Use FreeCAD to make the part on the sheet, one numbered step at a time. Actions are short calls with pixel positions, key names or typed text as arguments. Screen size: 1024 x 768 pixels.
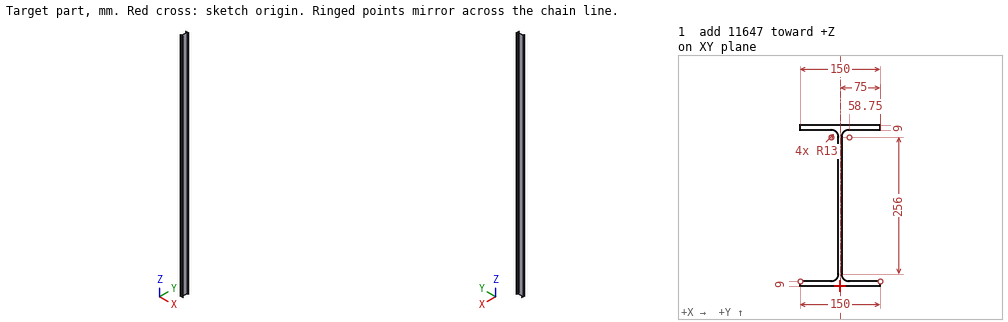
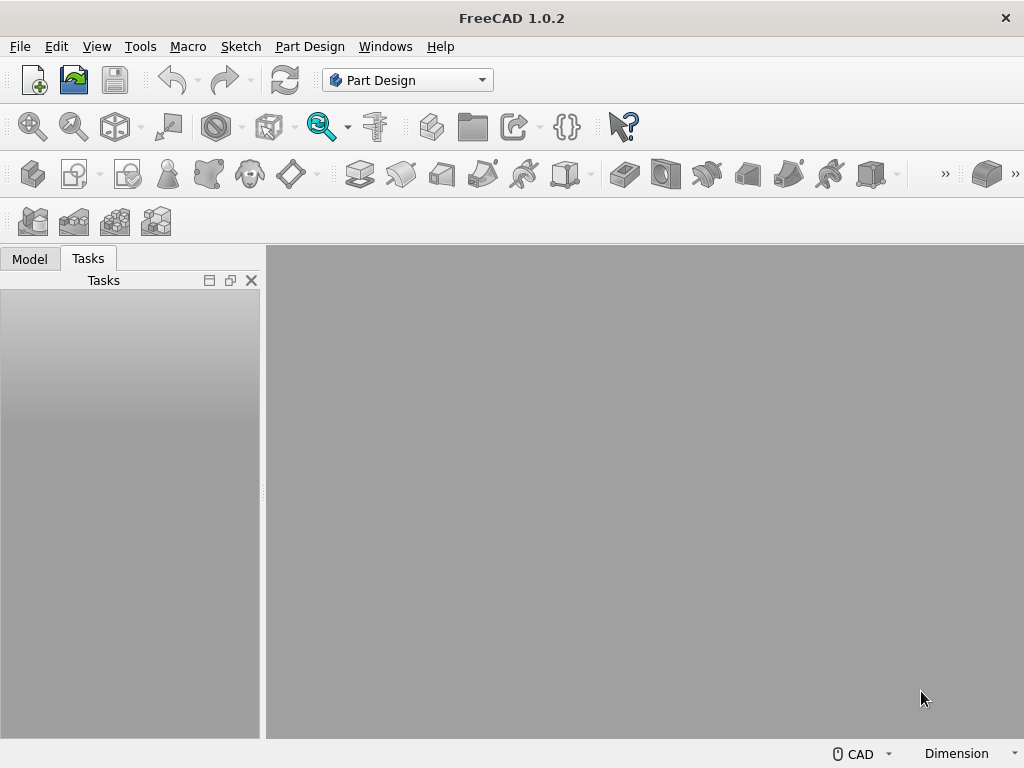
key(ctrl+n)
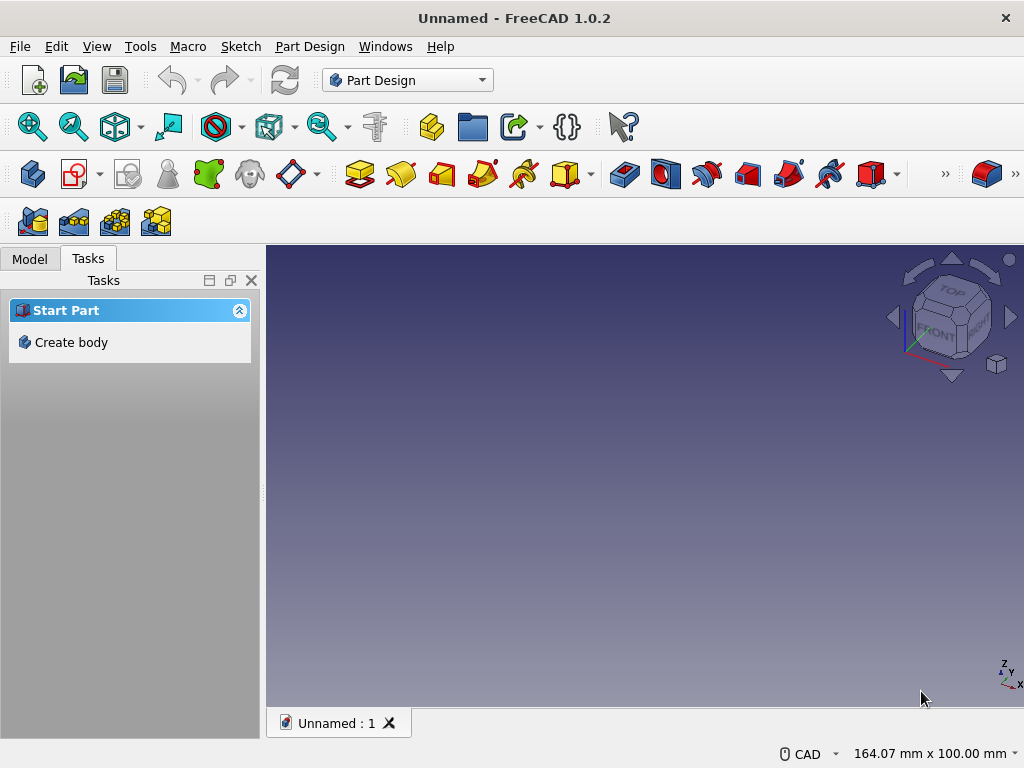
click(74, 174)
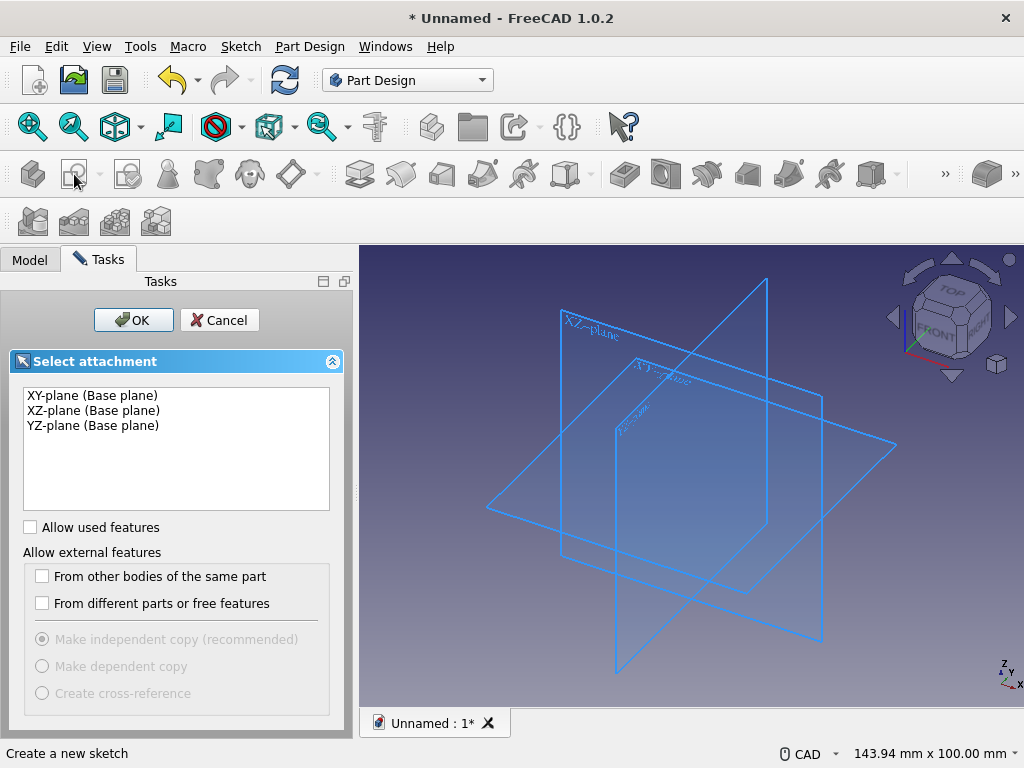
click(84, 396)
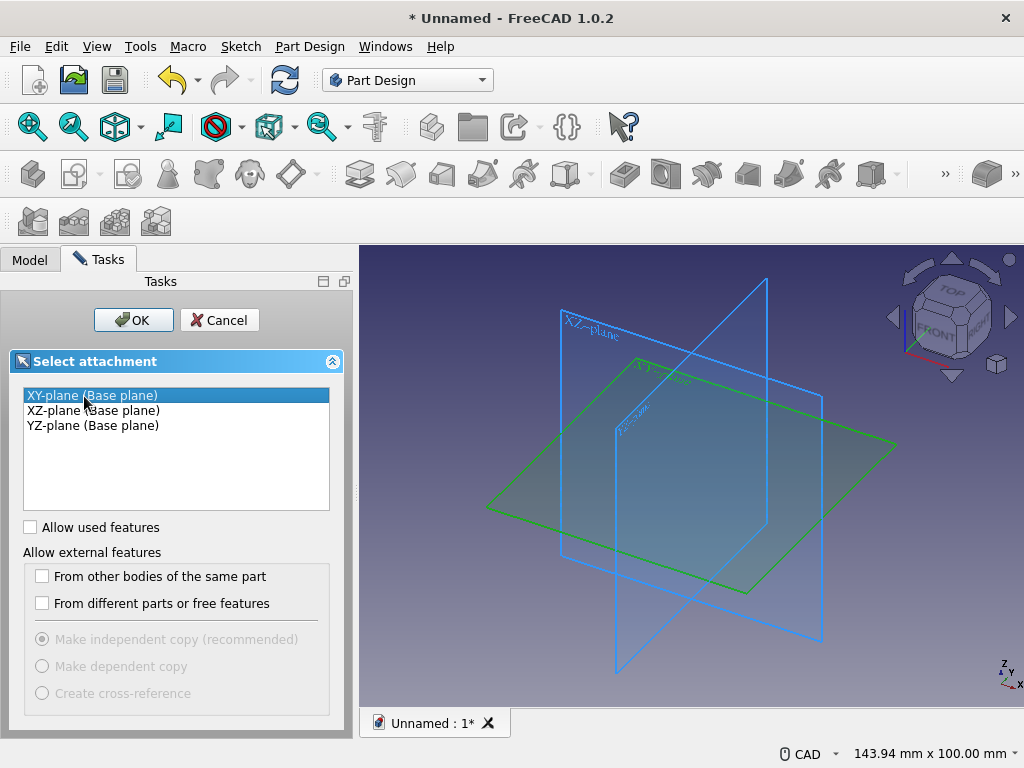
click(134, 320)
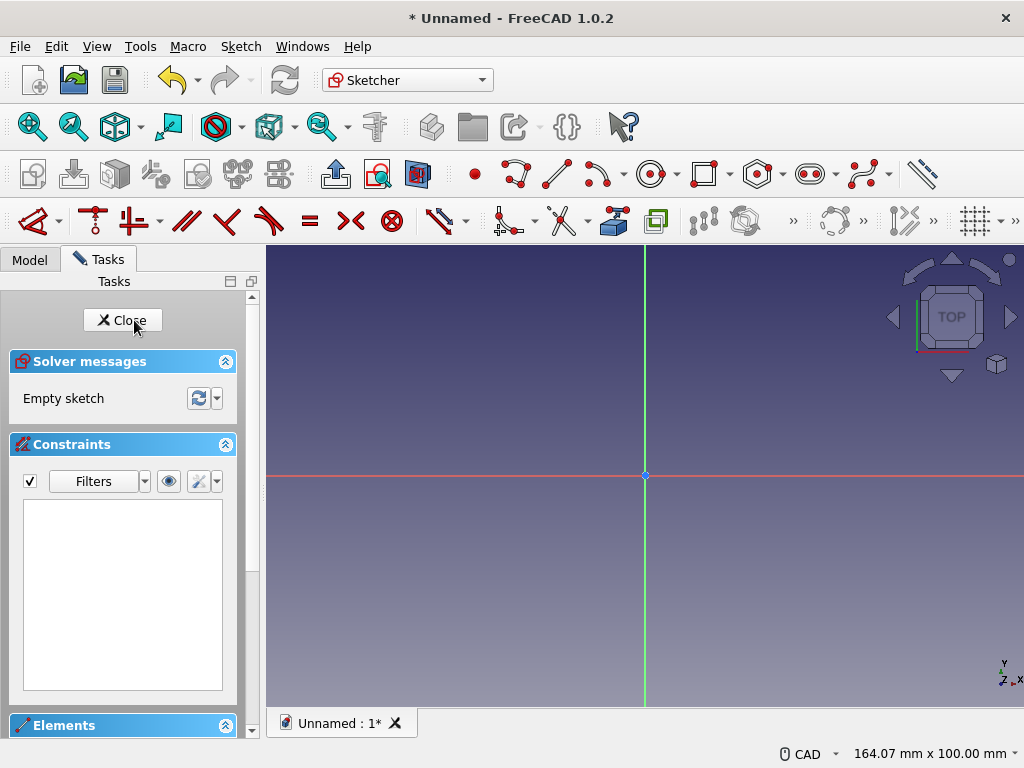
scroll(559, 651, down, 8)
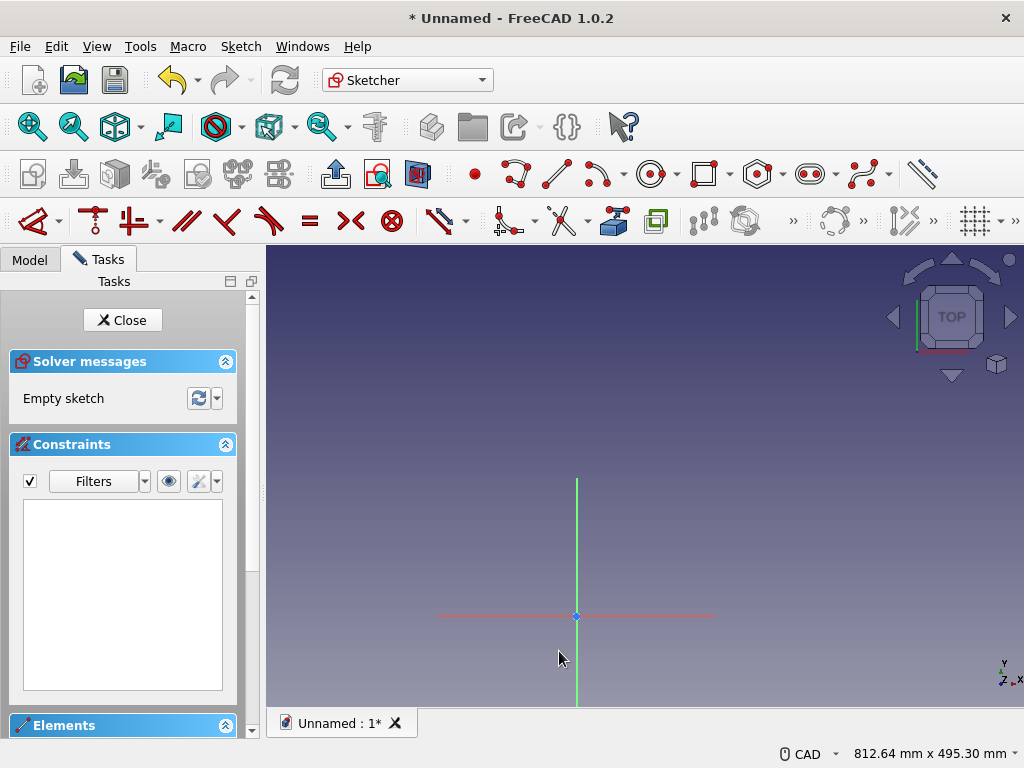
key(g)
key(l)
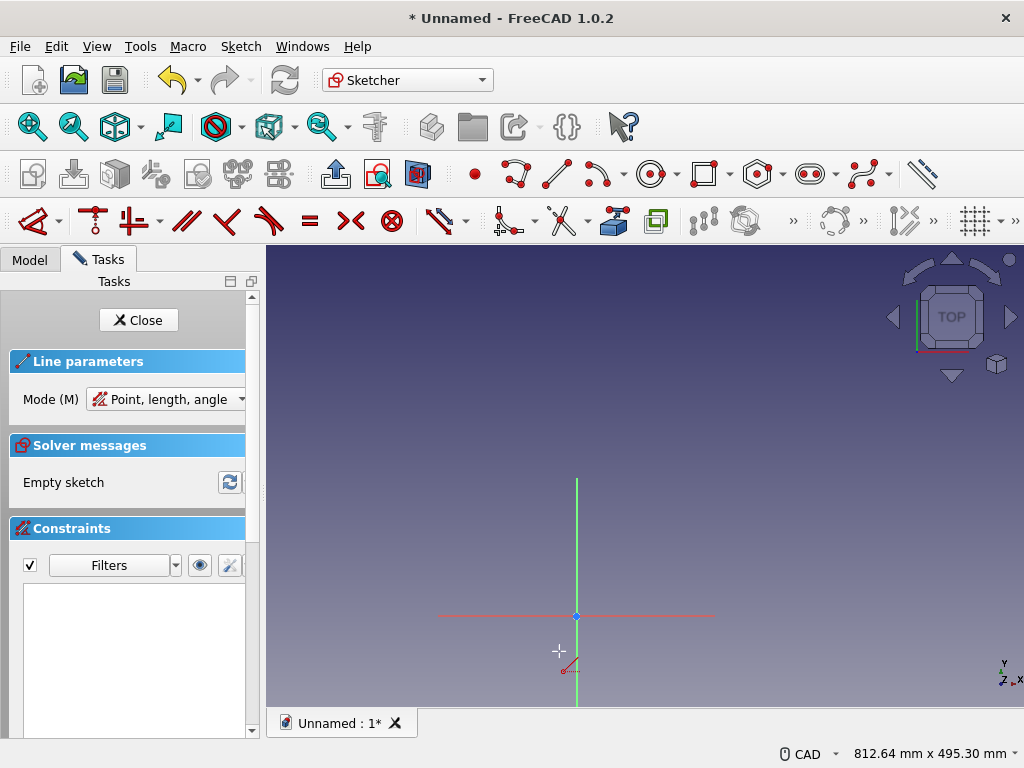
scroll(580, 596, up, 9)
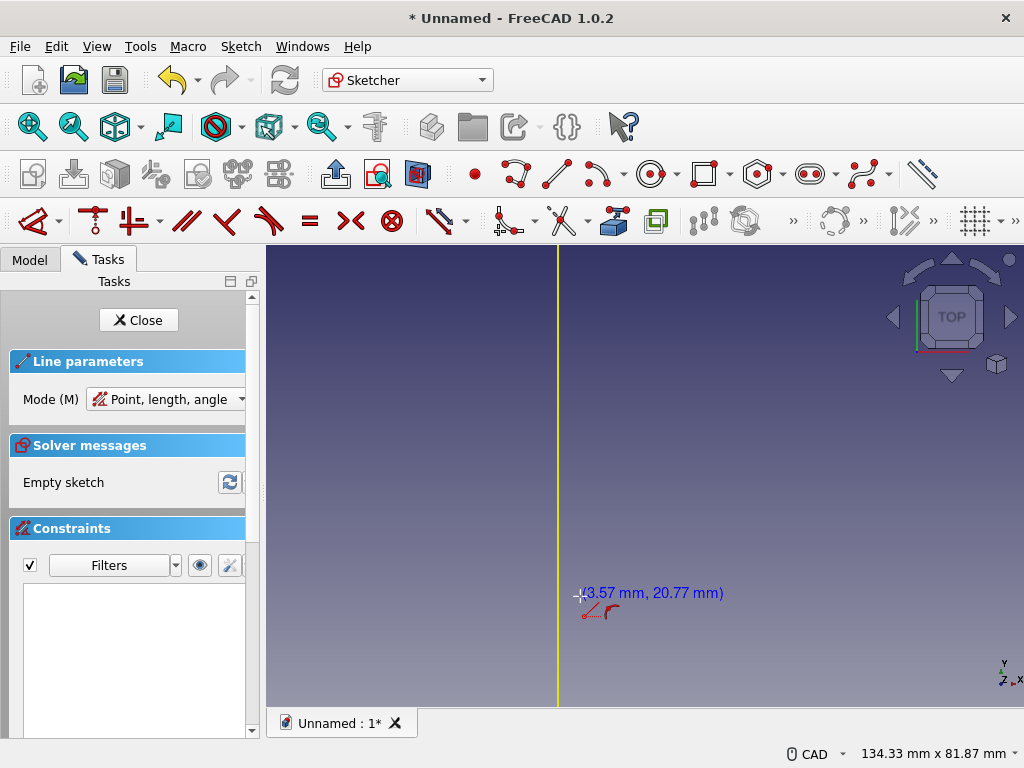
click(576, 591)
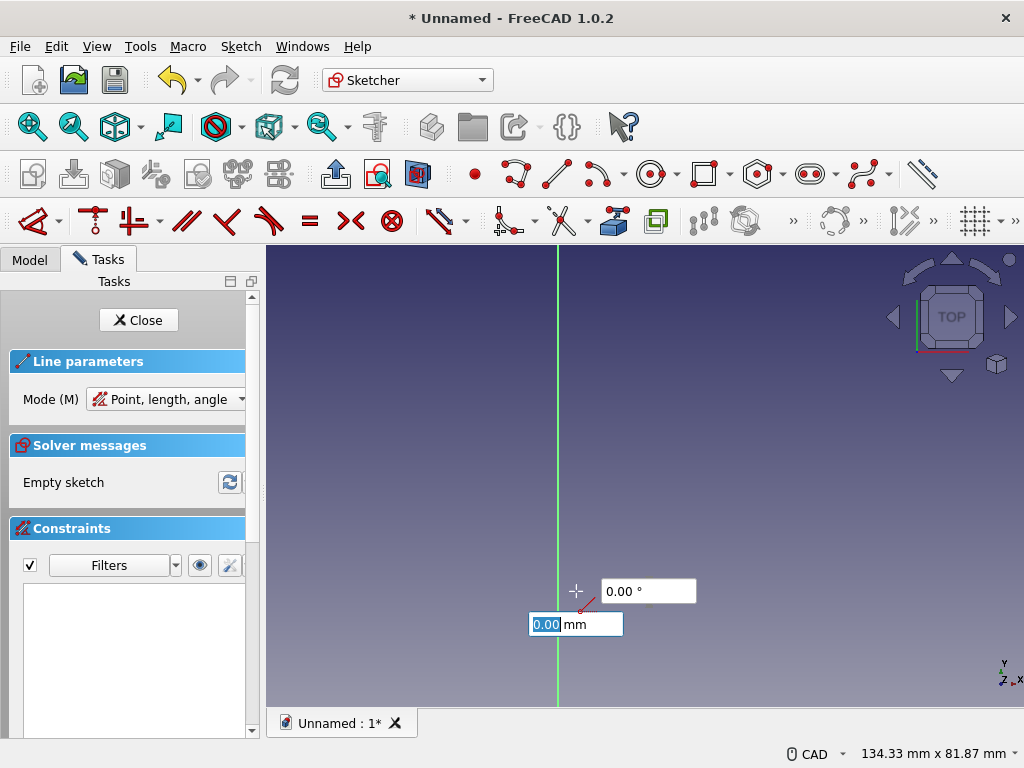
scroll(580, 596, down, 9)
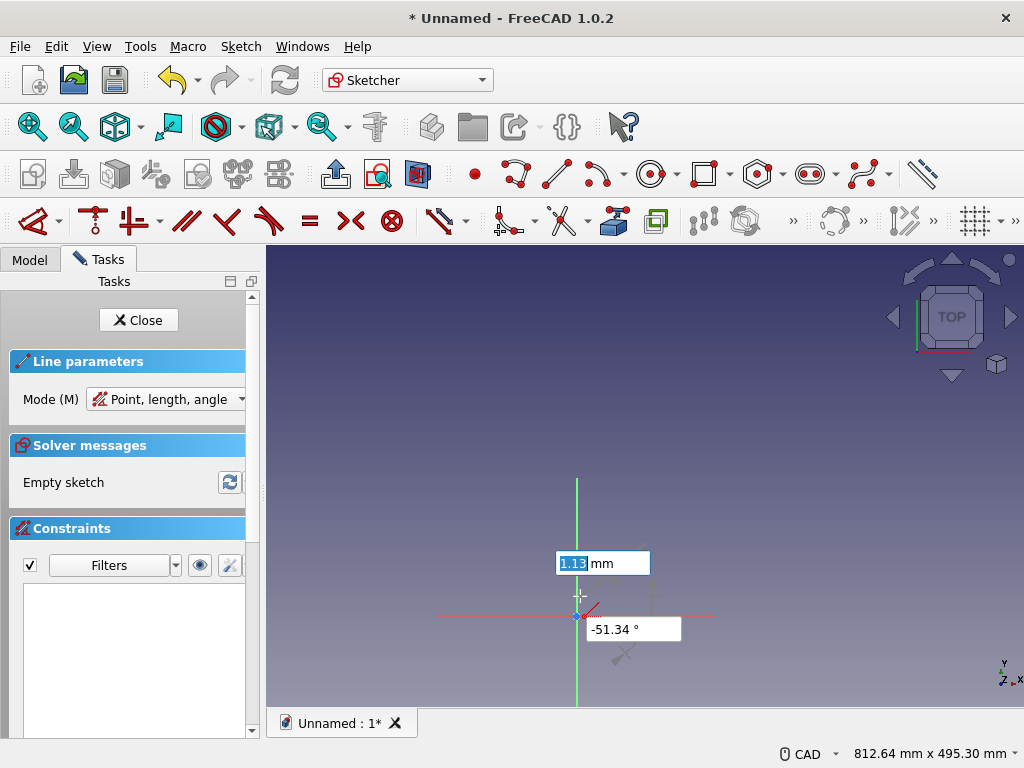
scroll(580, 357, up, 9)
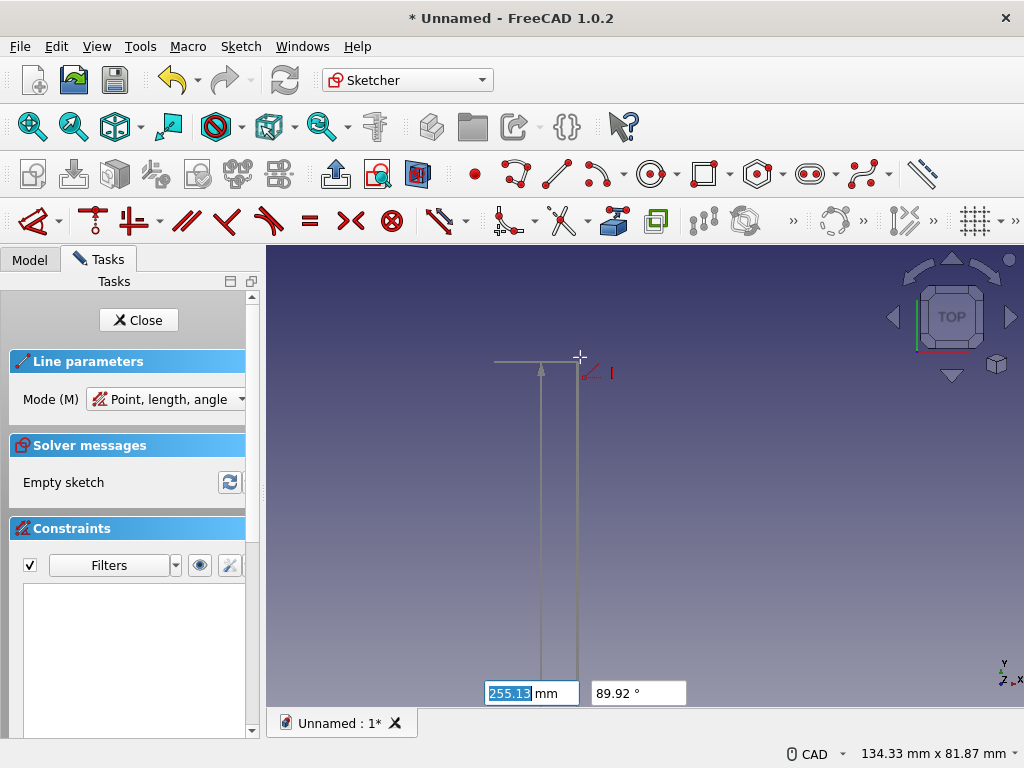
click(576, 356)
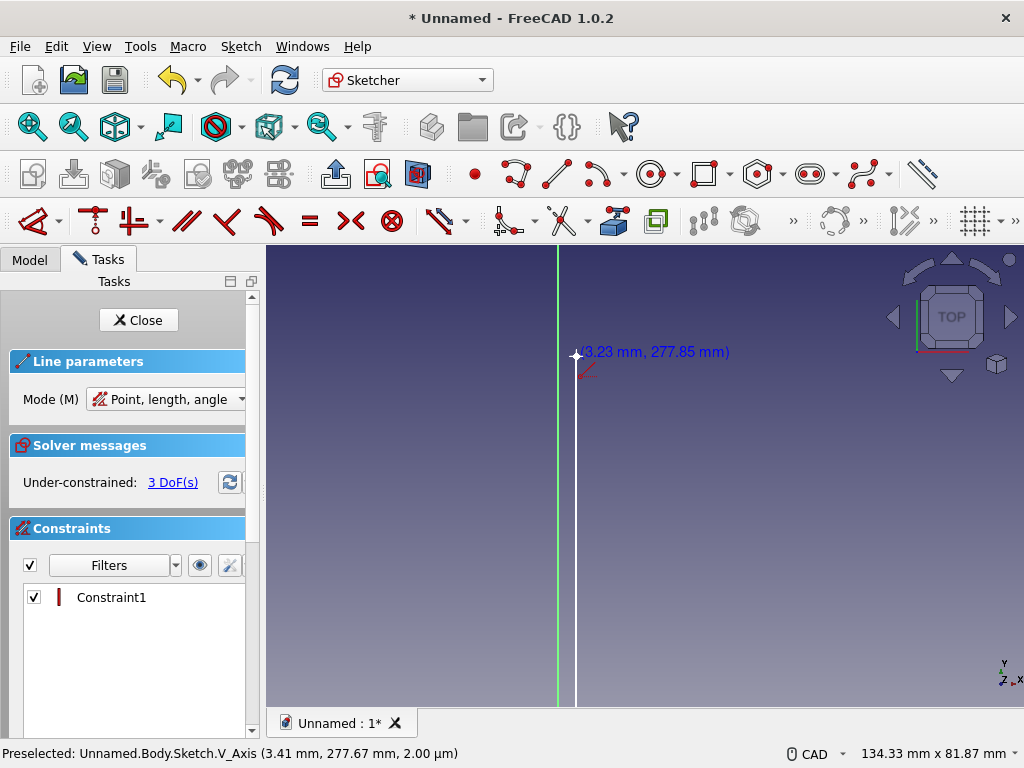
key(g)
key(m)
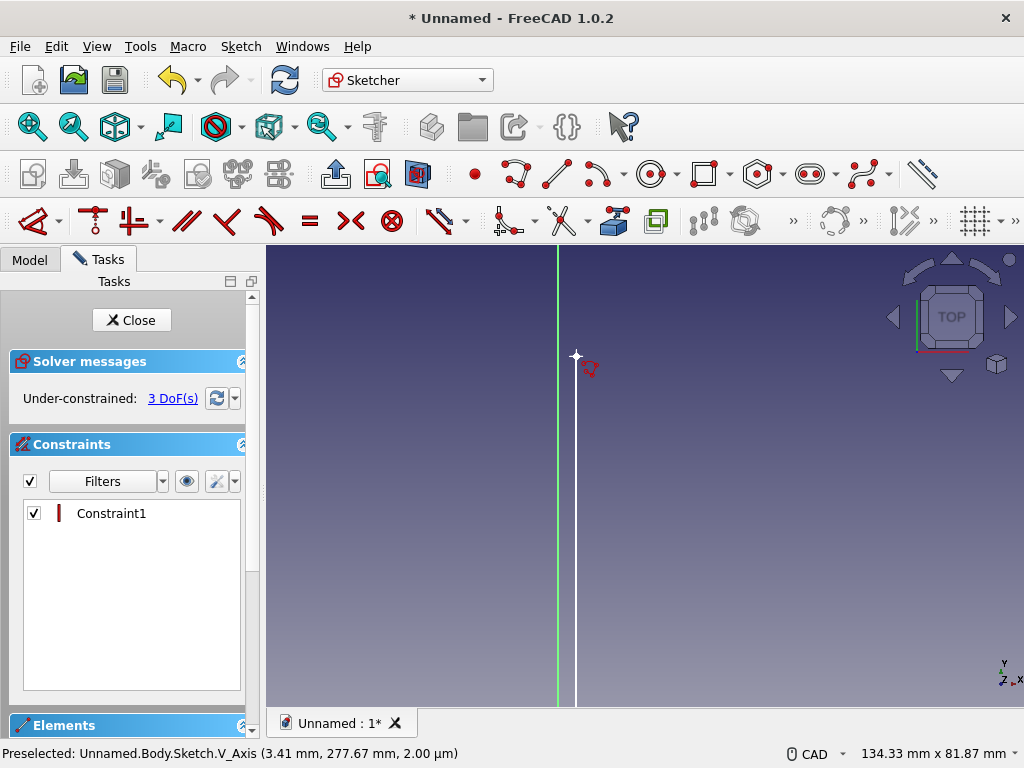
scroll(580, 357, down, 9)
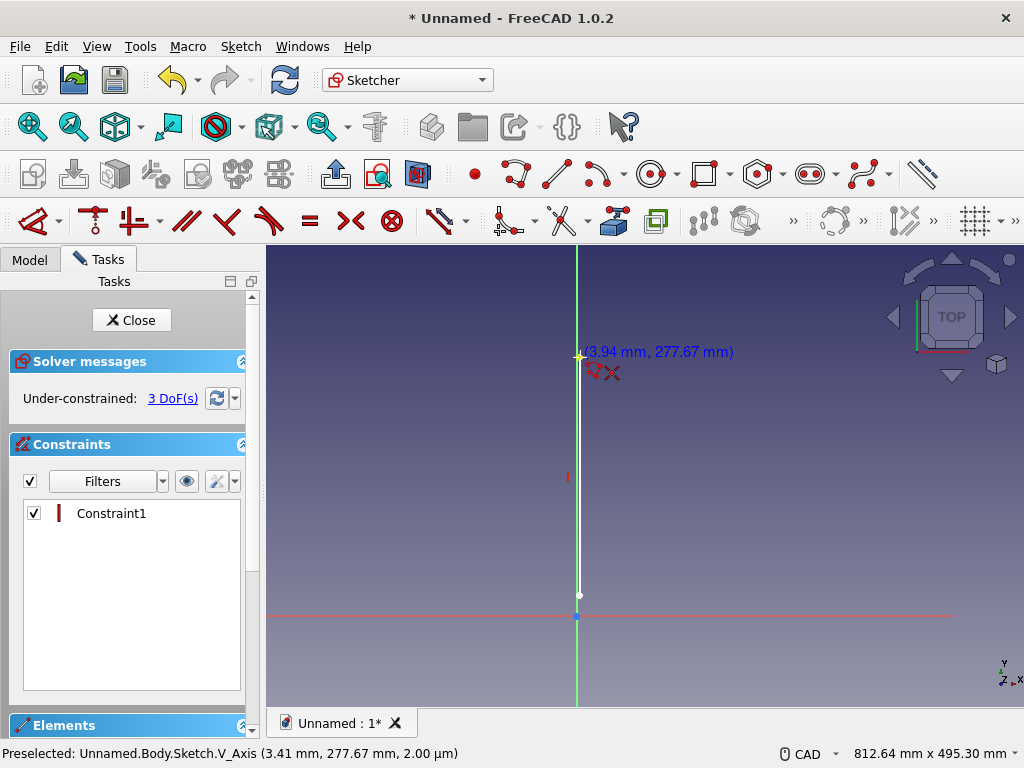
click(592, 345)
click(647, 345)